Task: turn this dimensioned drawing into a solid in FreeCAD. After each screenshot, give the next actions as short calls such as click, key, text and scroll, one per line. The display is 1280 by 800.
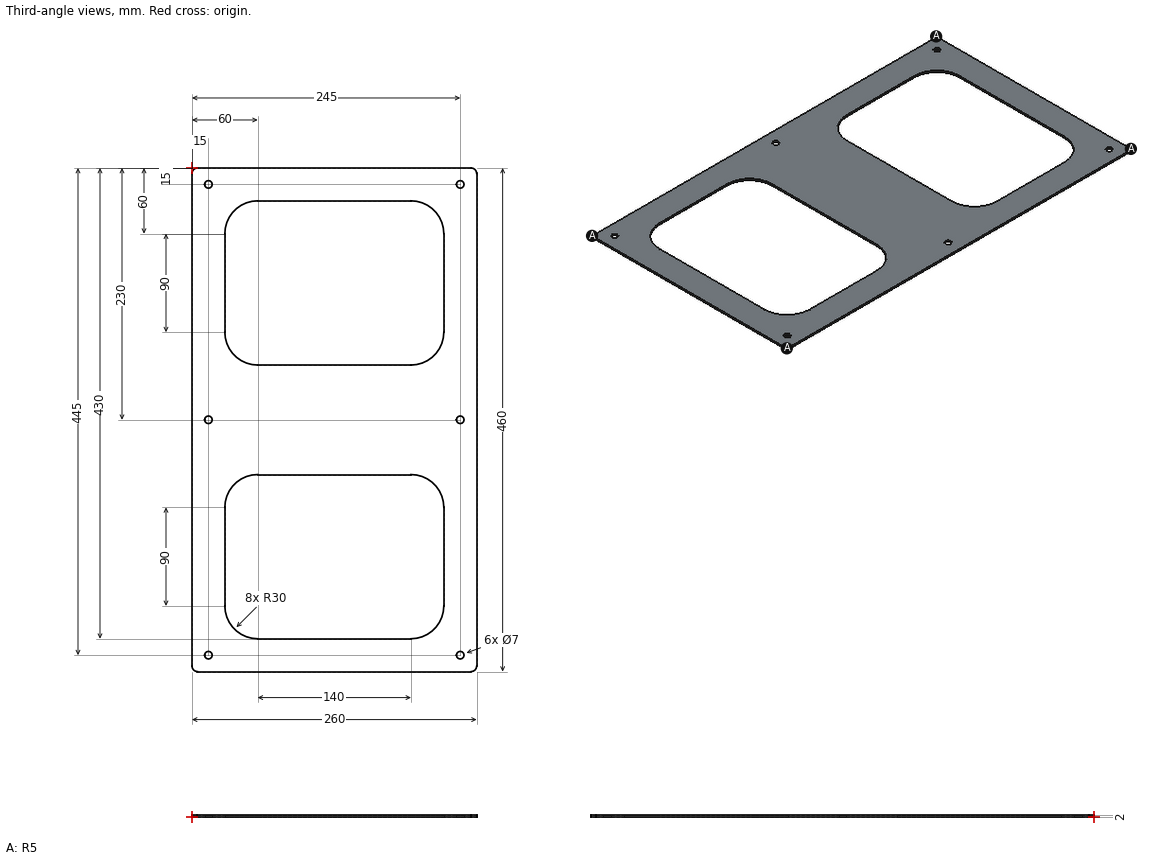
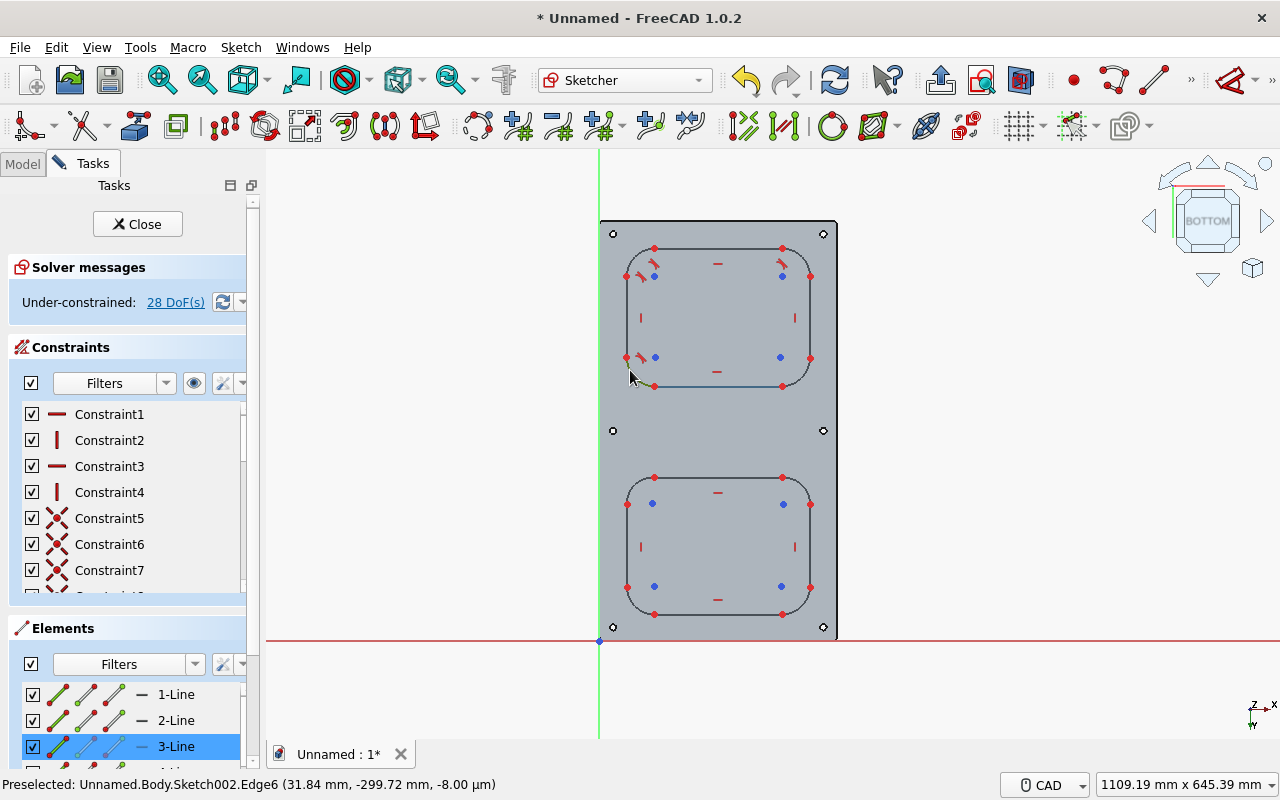
key(t)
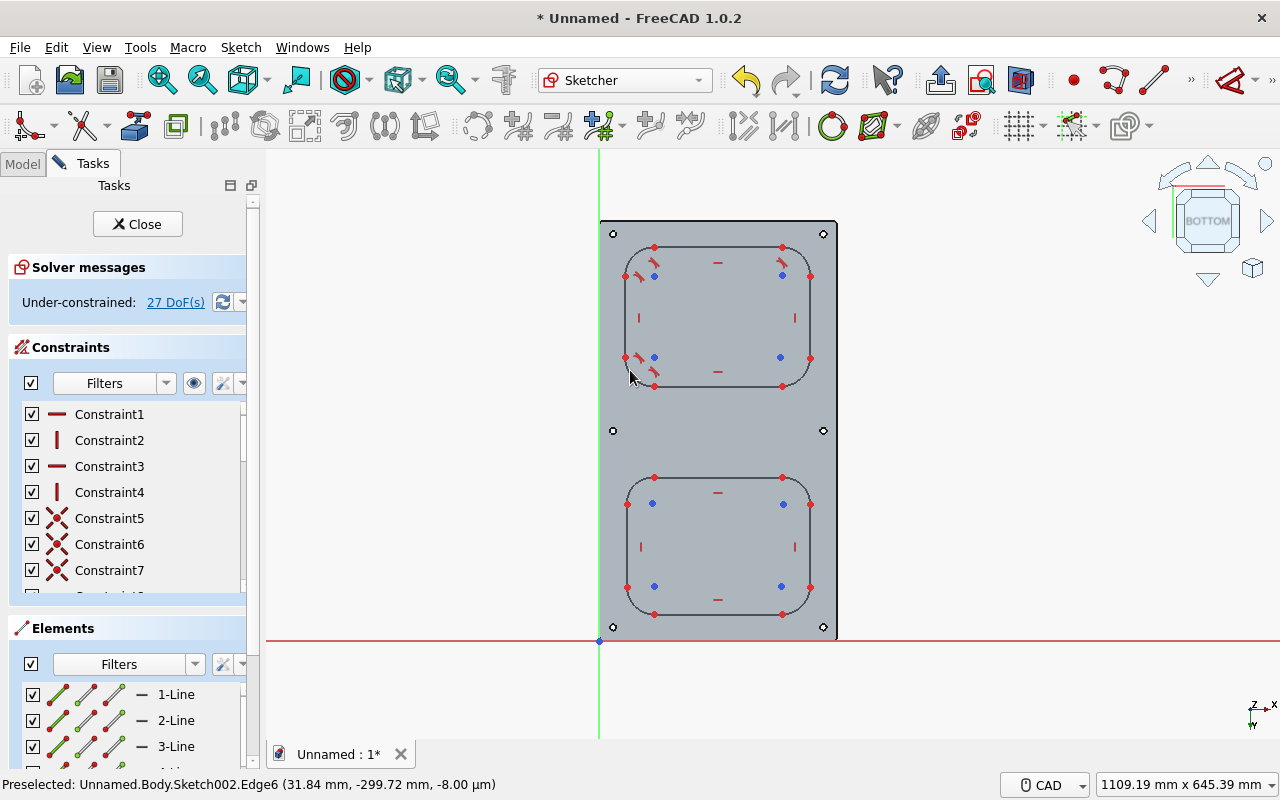
click(692, 387)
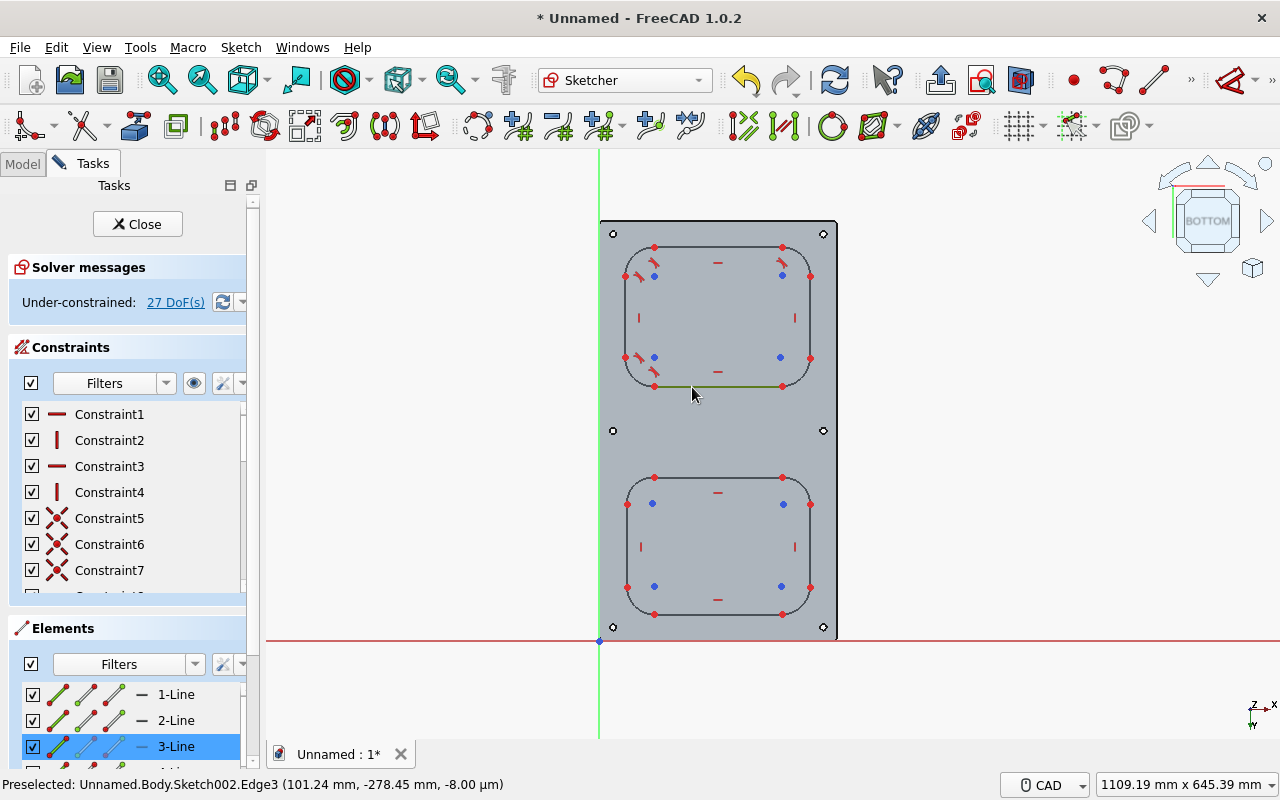
click(794, 383)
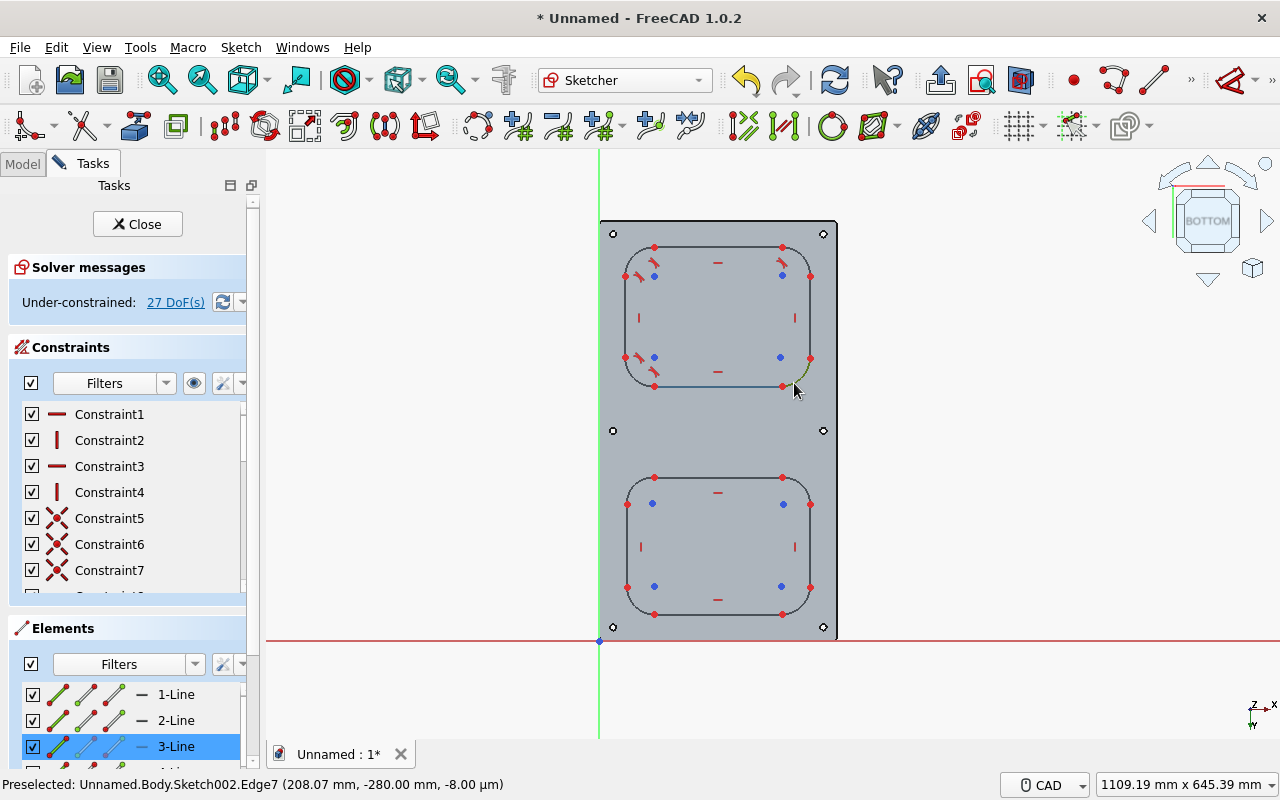
key(t)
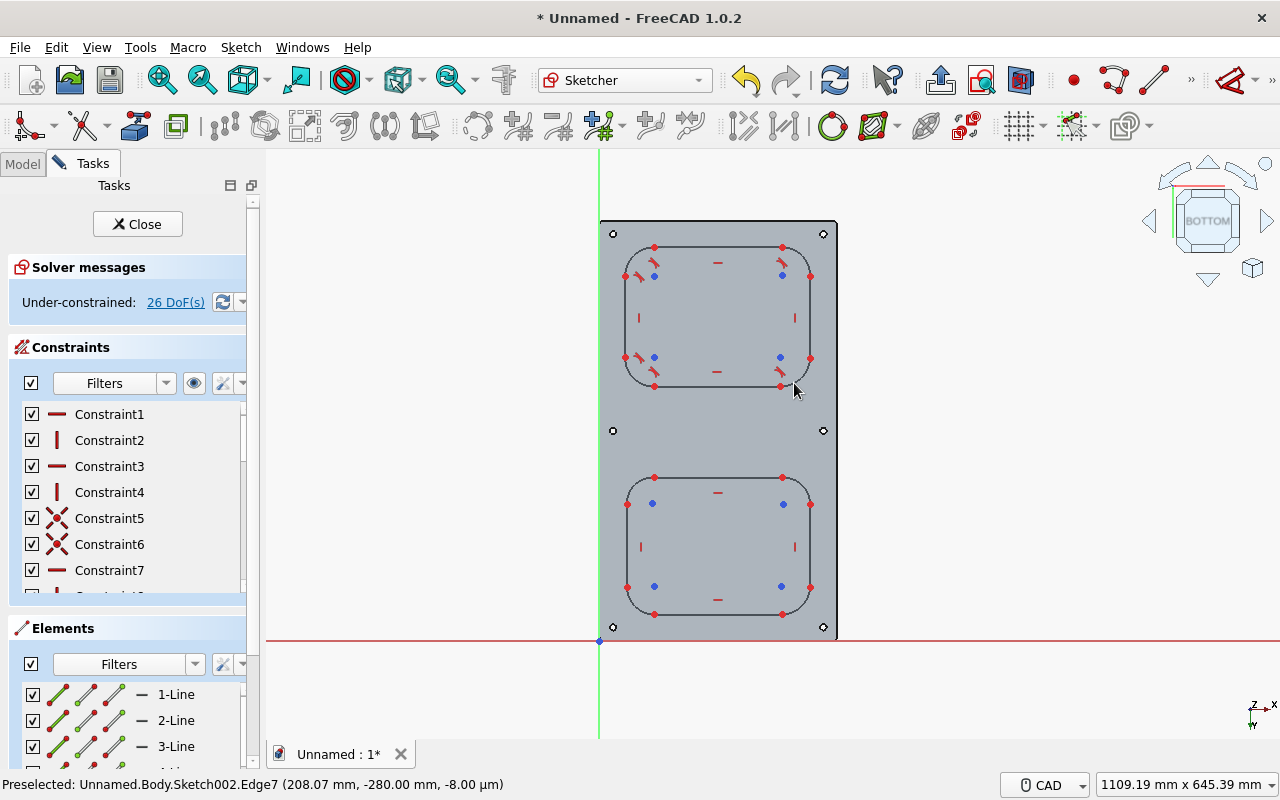
click(810, 334)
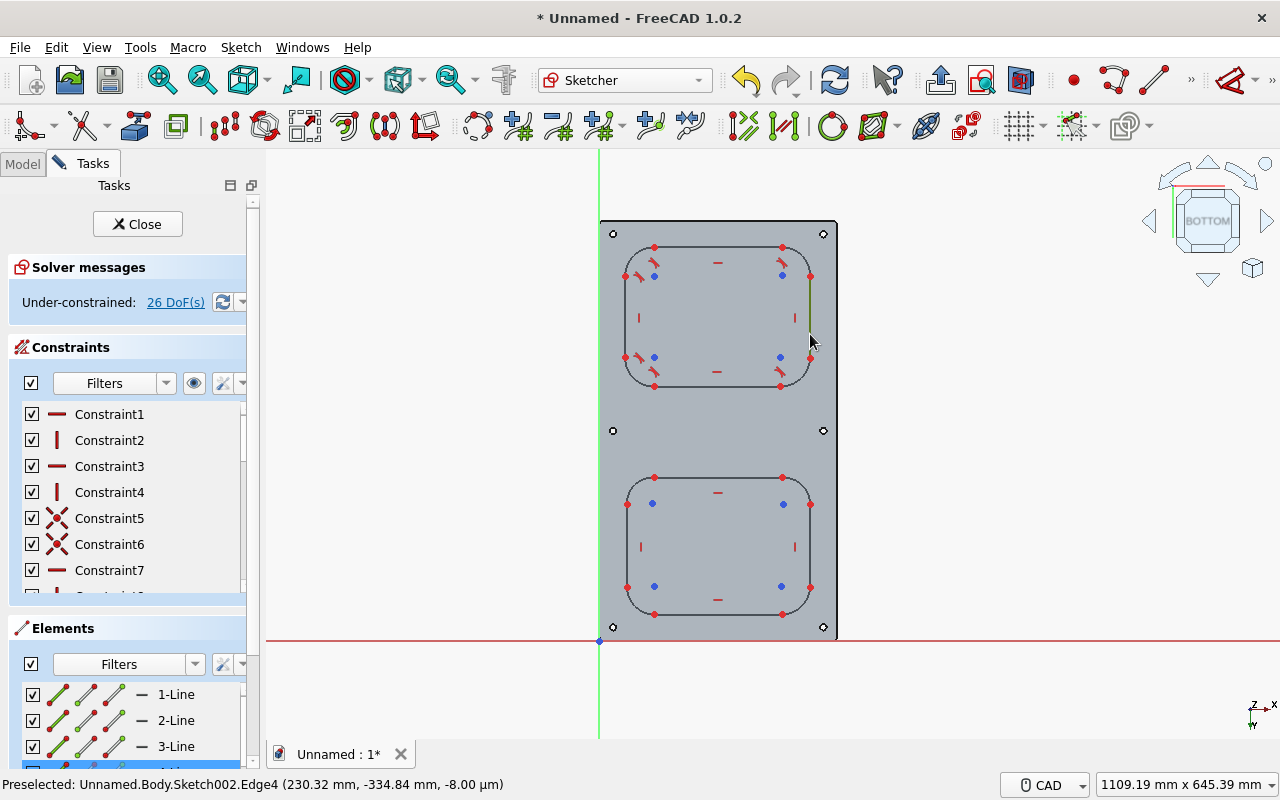
click(794, 384)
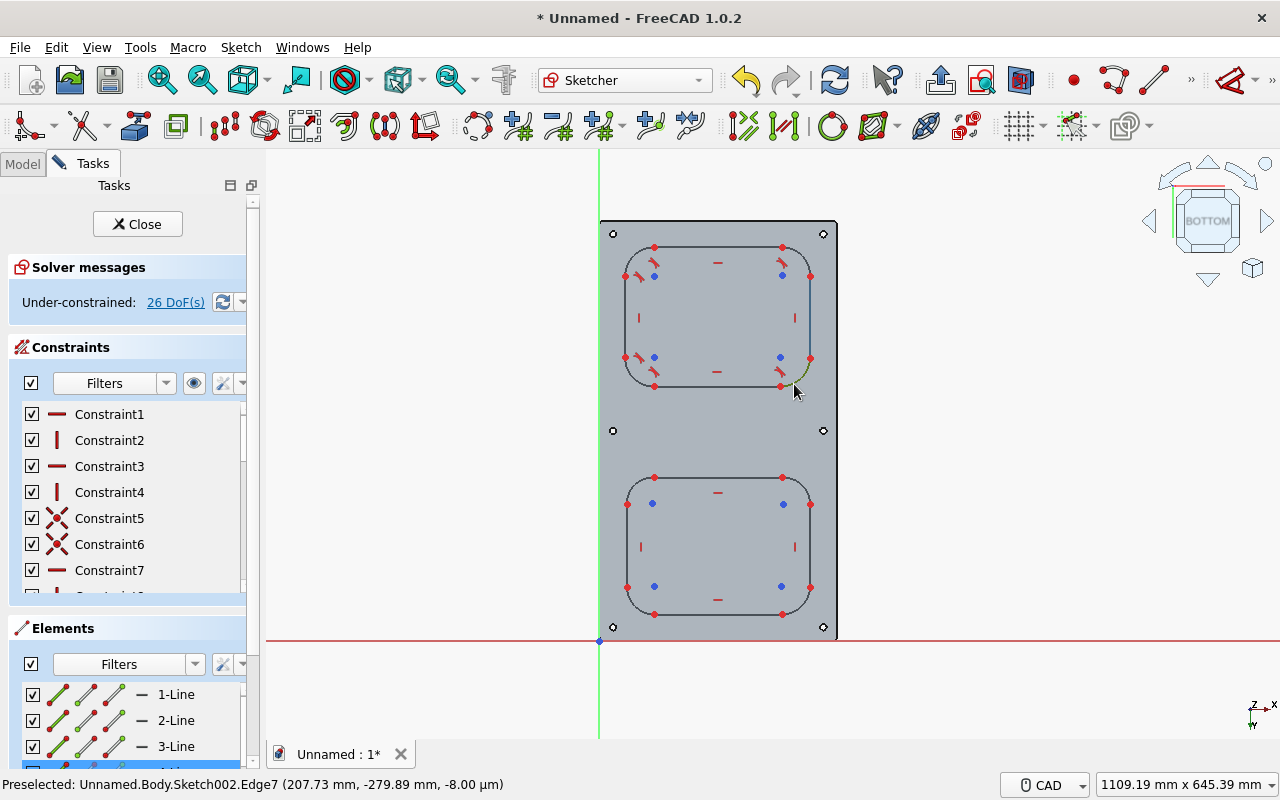
key(t)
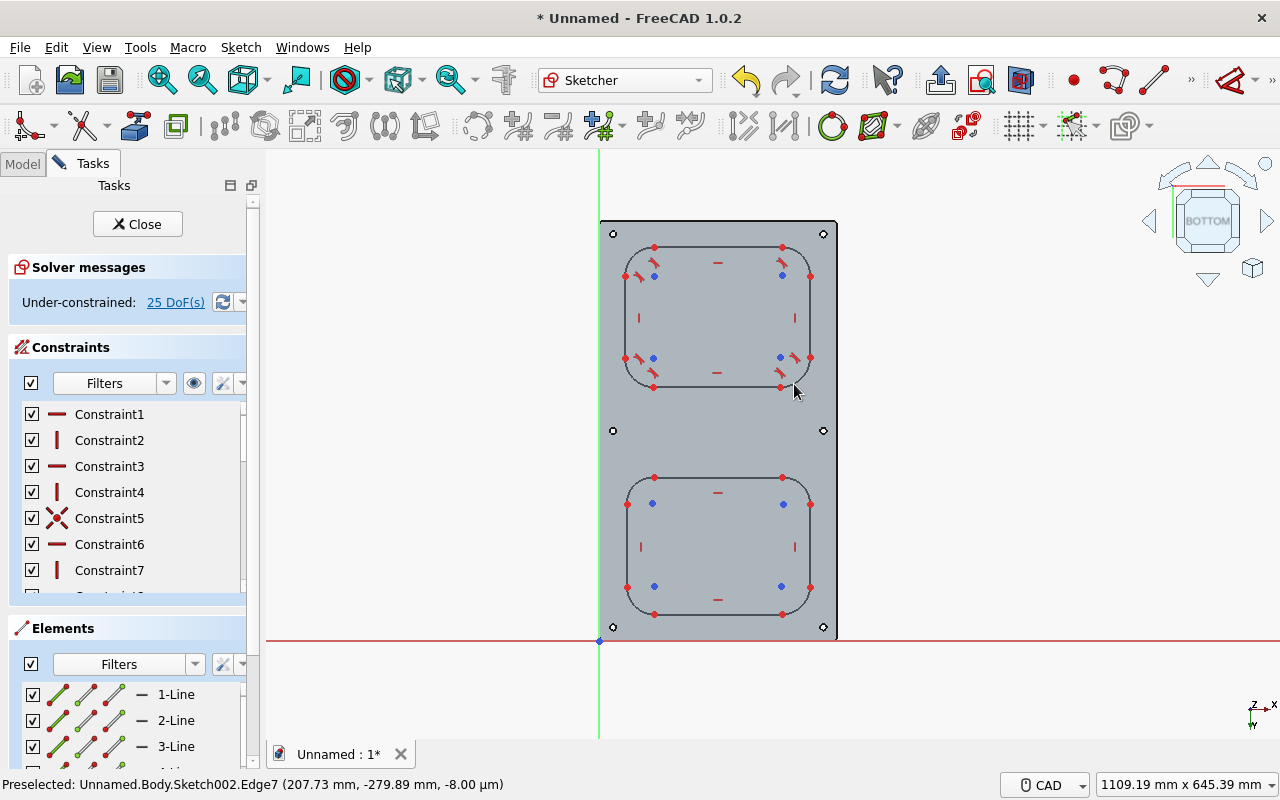
click(810, 333)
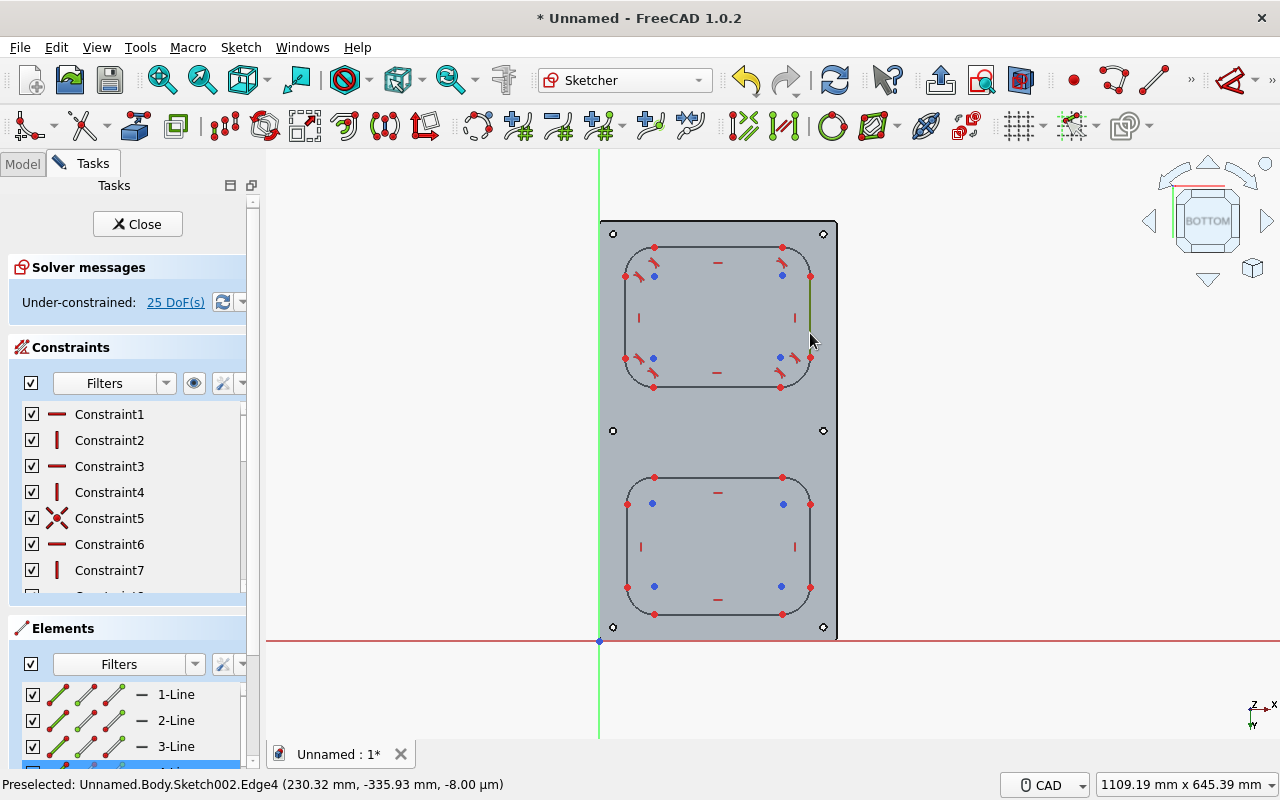
click(807, 263)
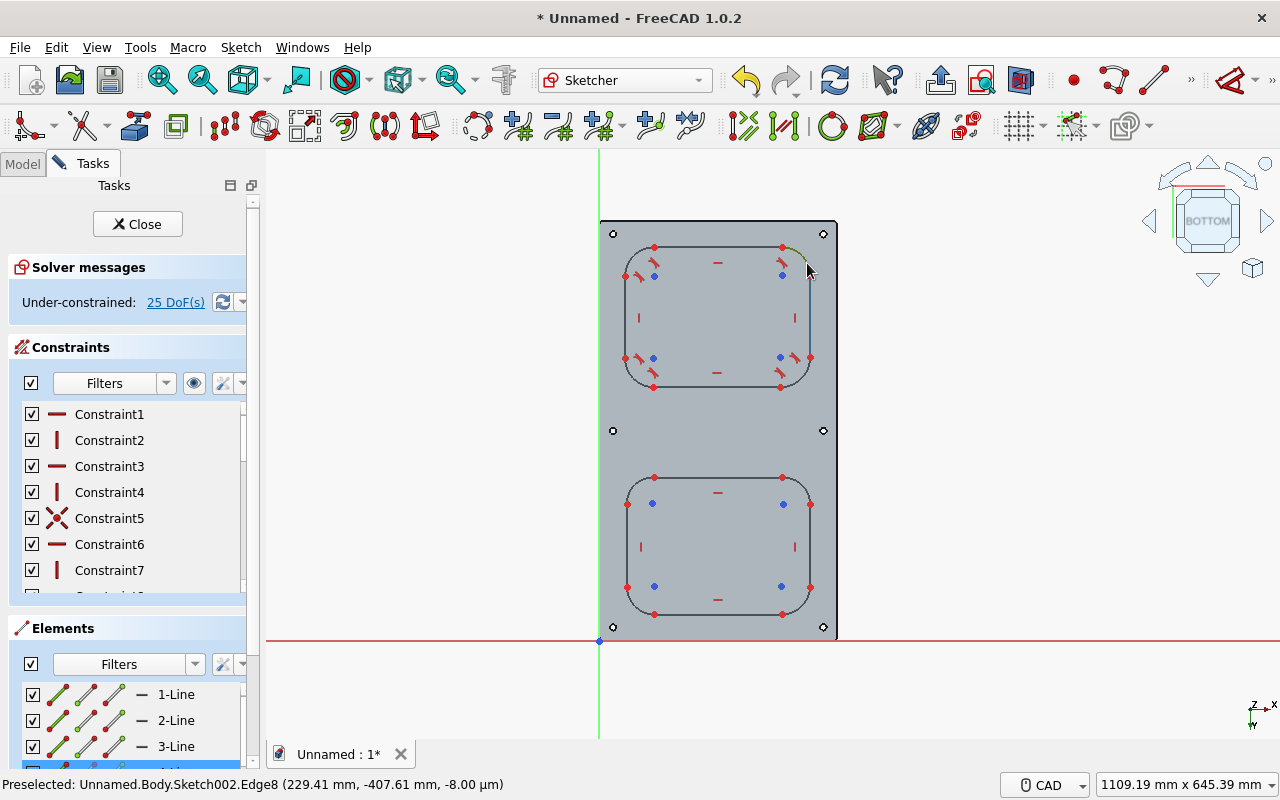
key(t)